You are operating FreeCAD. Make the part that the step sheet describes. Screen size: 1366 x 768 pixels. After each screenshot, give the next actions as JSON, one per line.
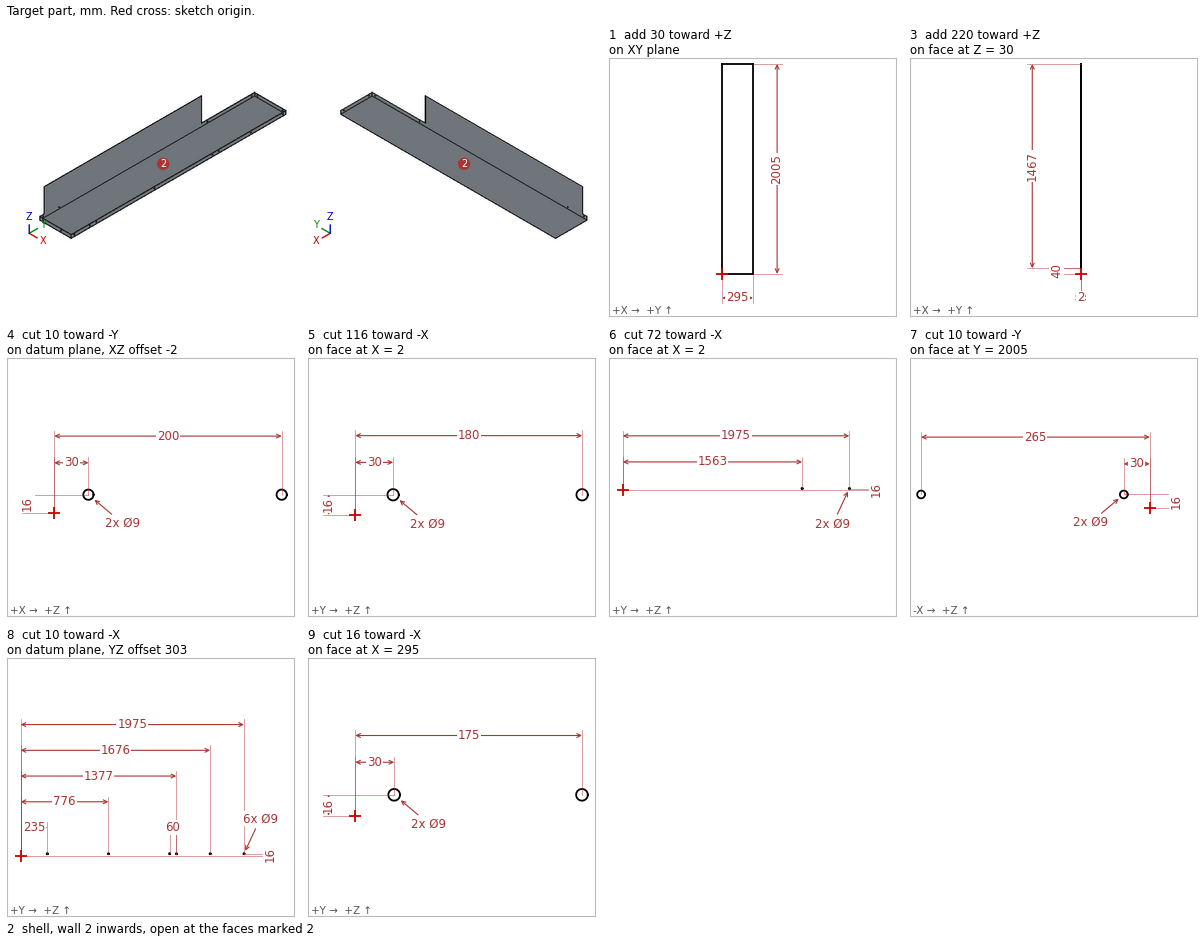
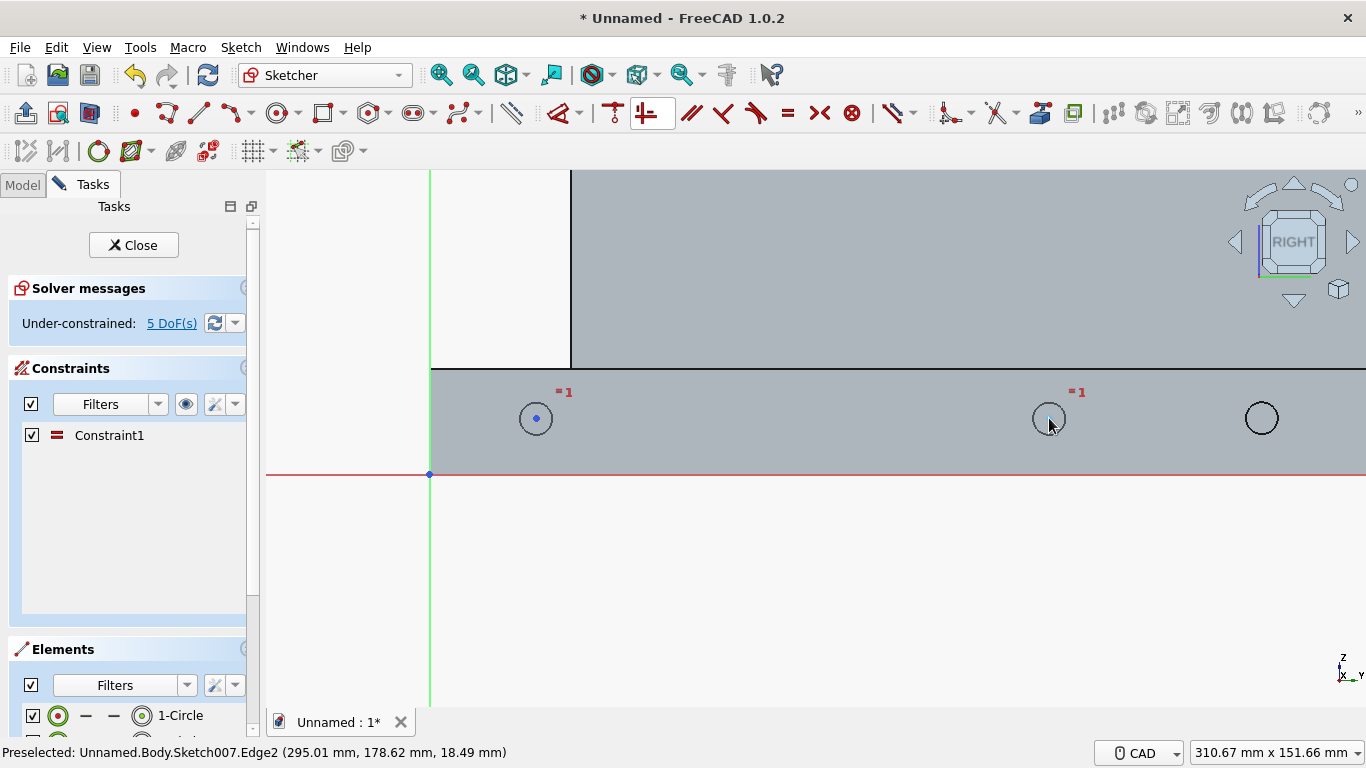
{"action": "left_click", "coordinate": [536, 419]}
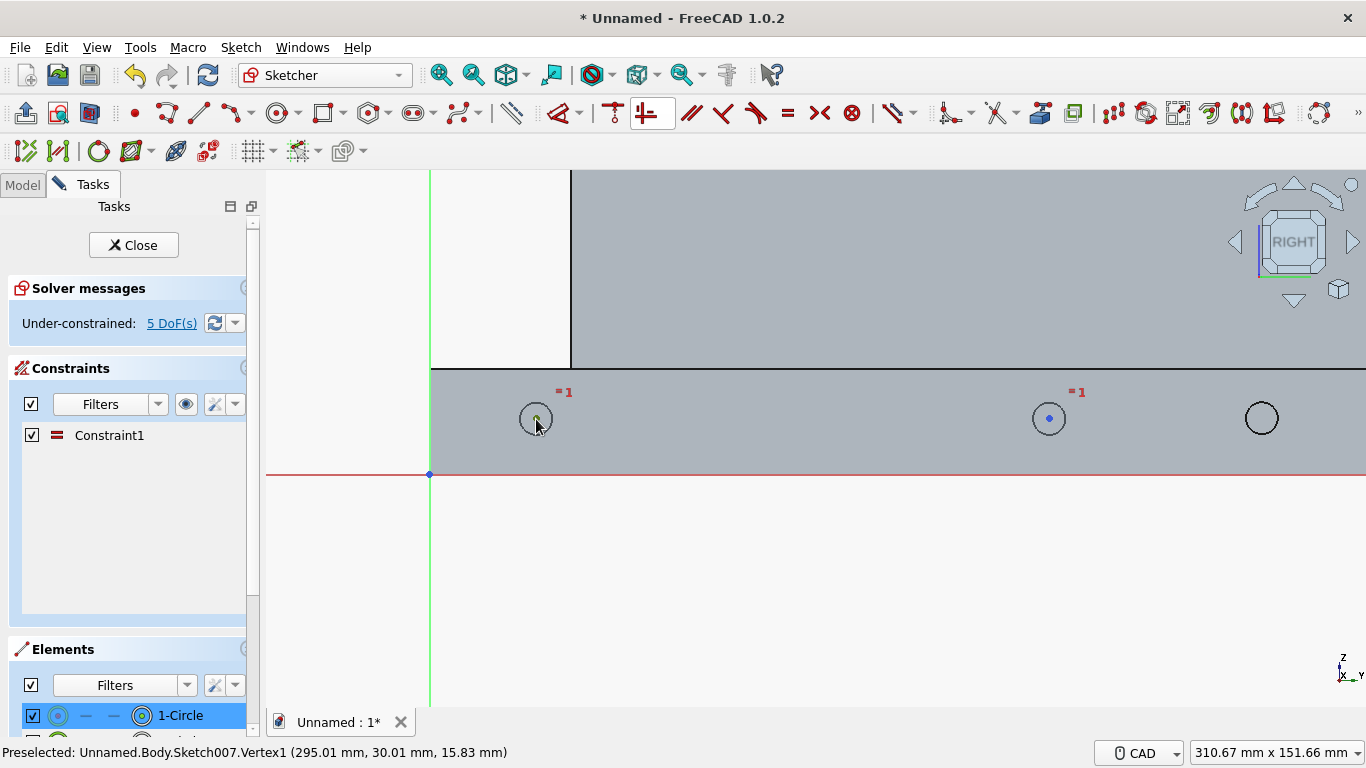
{"action": "left_click", "coordinate": [1049, 419]}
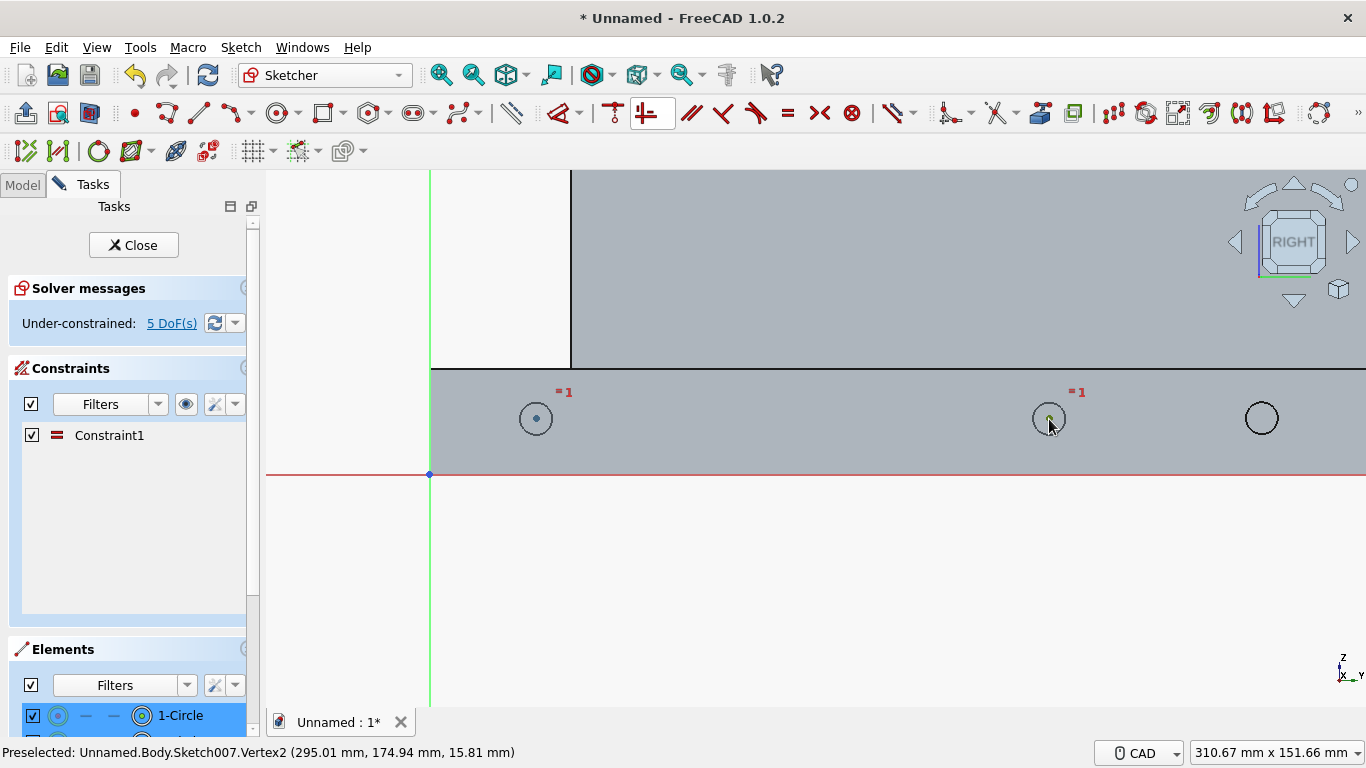
{"action": "left_click", "coordinate": [670, 114]}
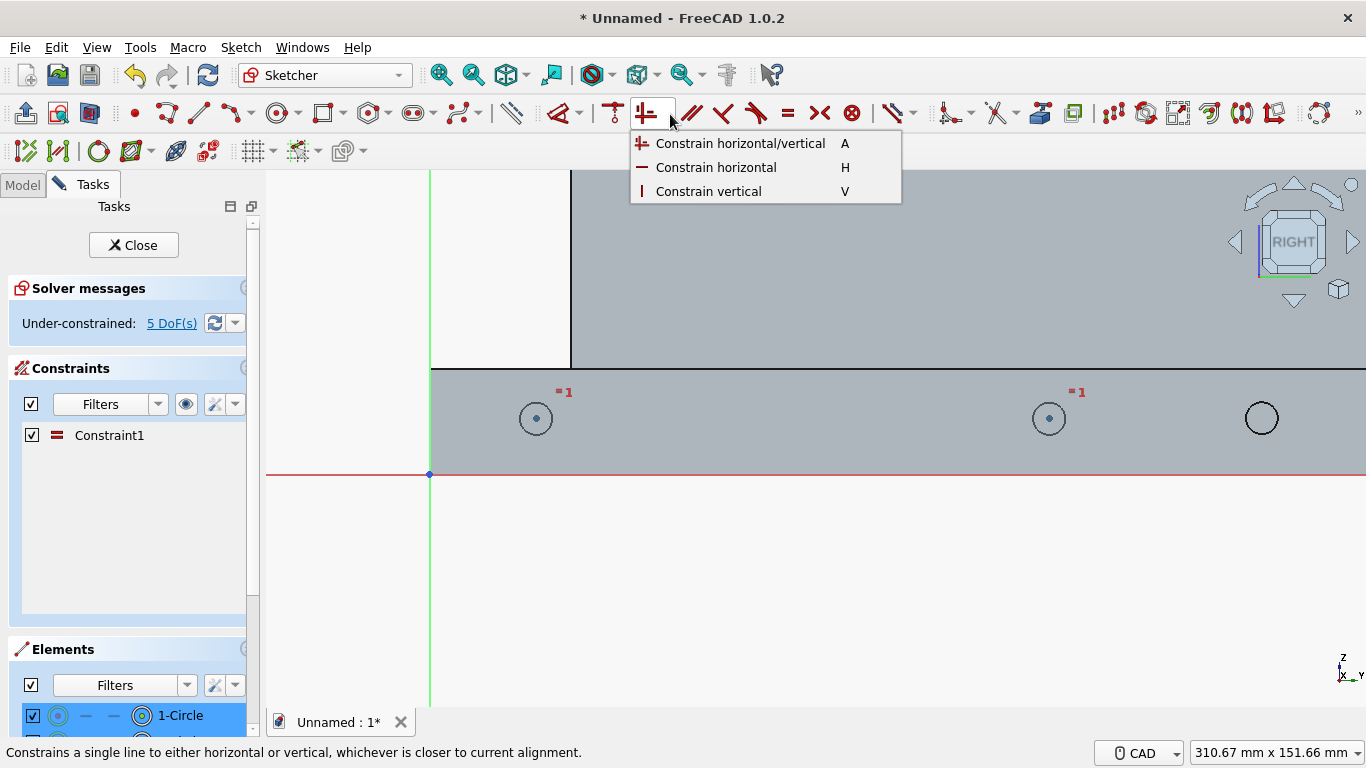
{"action": "left_click", "coordinate": [766, 167]}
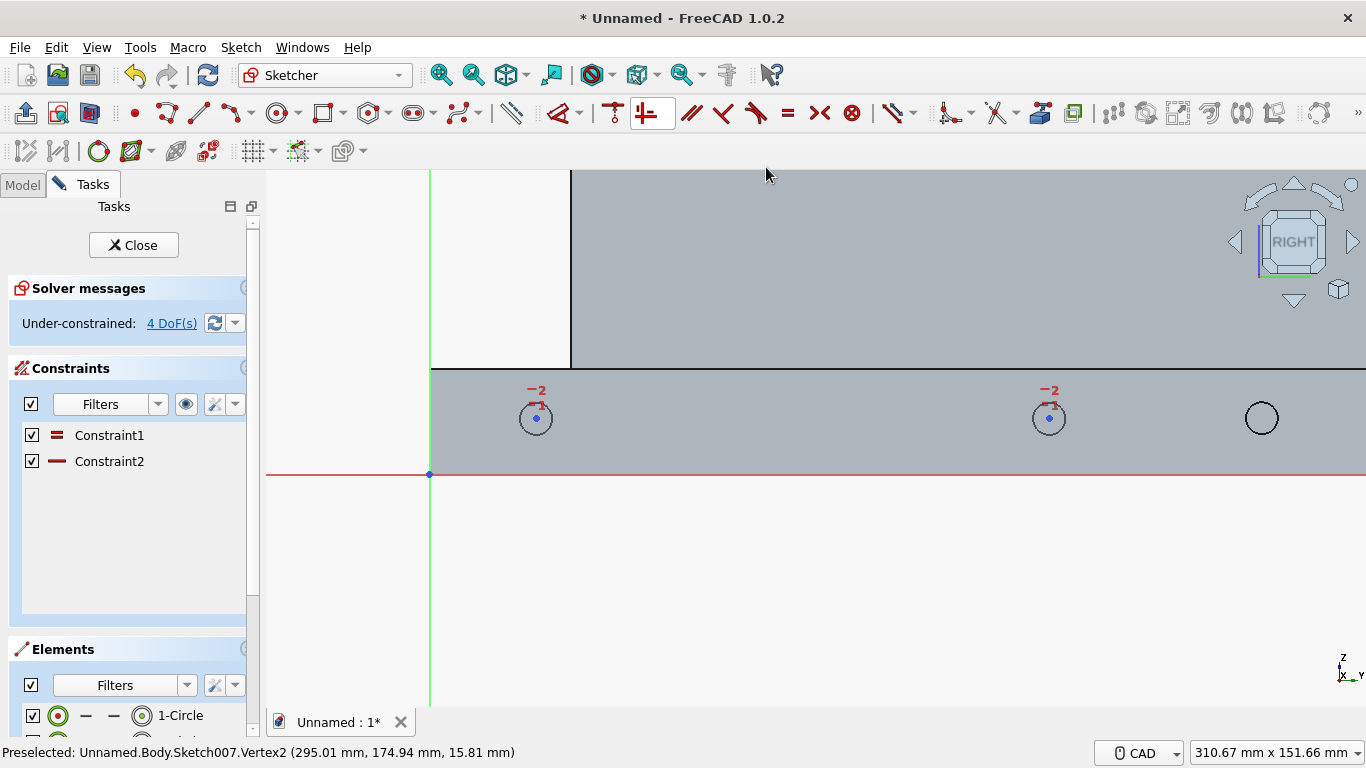
{"action": "left_click", "coordinate": [558, 114]}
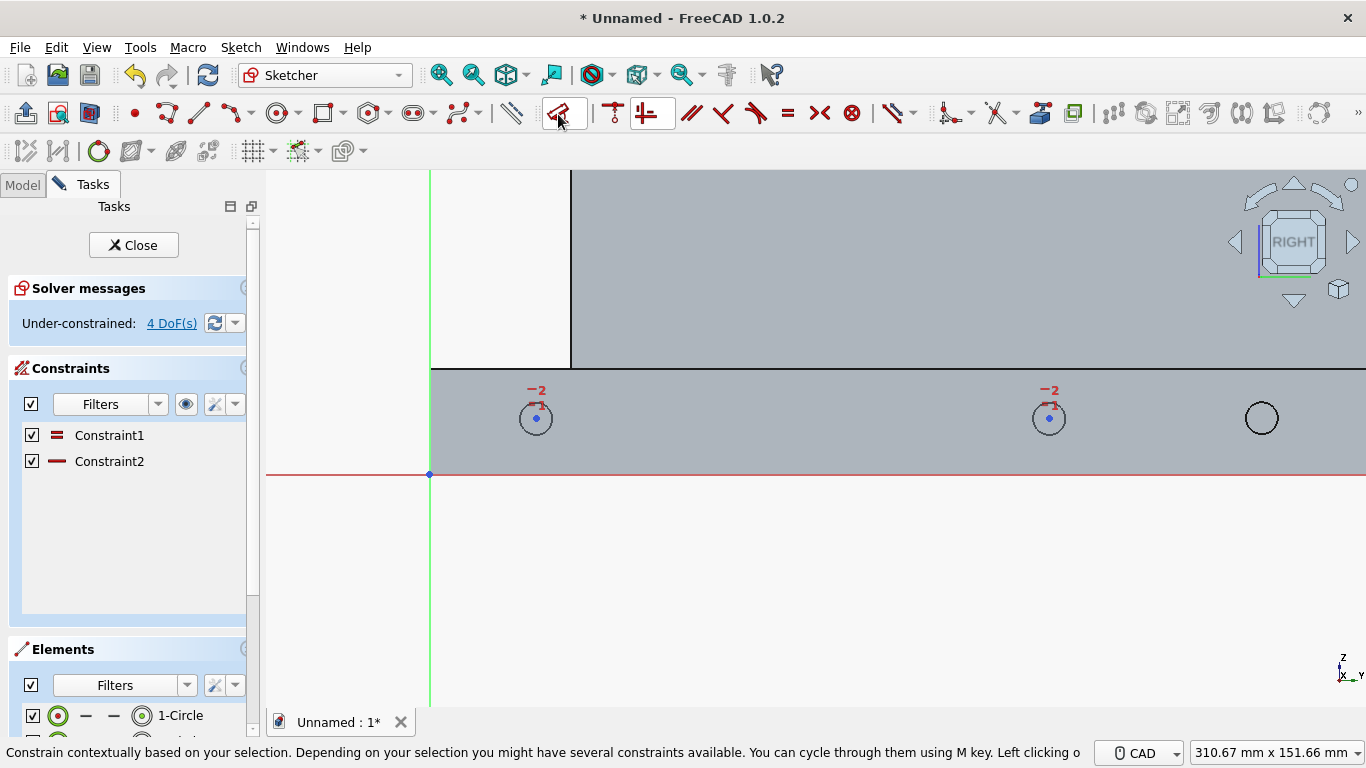
{"action": "scroll", "coordinate": [547, 407], "scroll_direction": "up", "scroll_amount": 2}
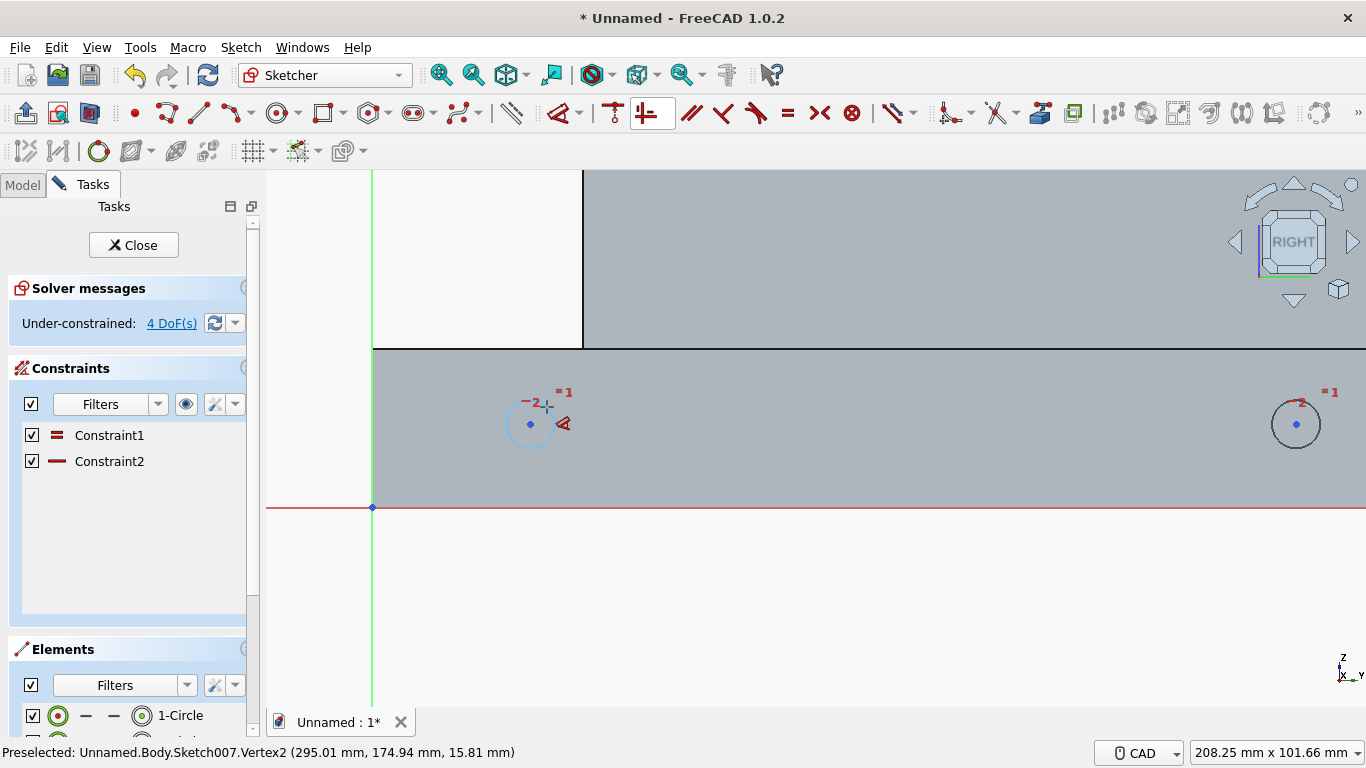
{"action": "left_click", "coordinate": [548, 407]}
{"action": "left_click", "coordinate": [571, 384]}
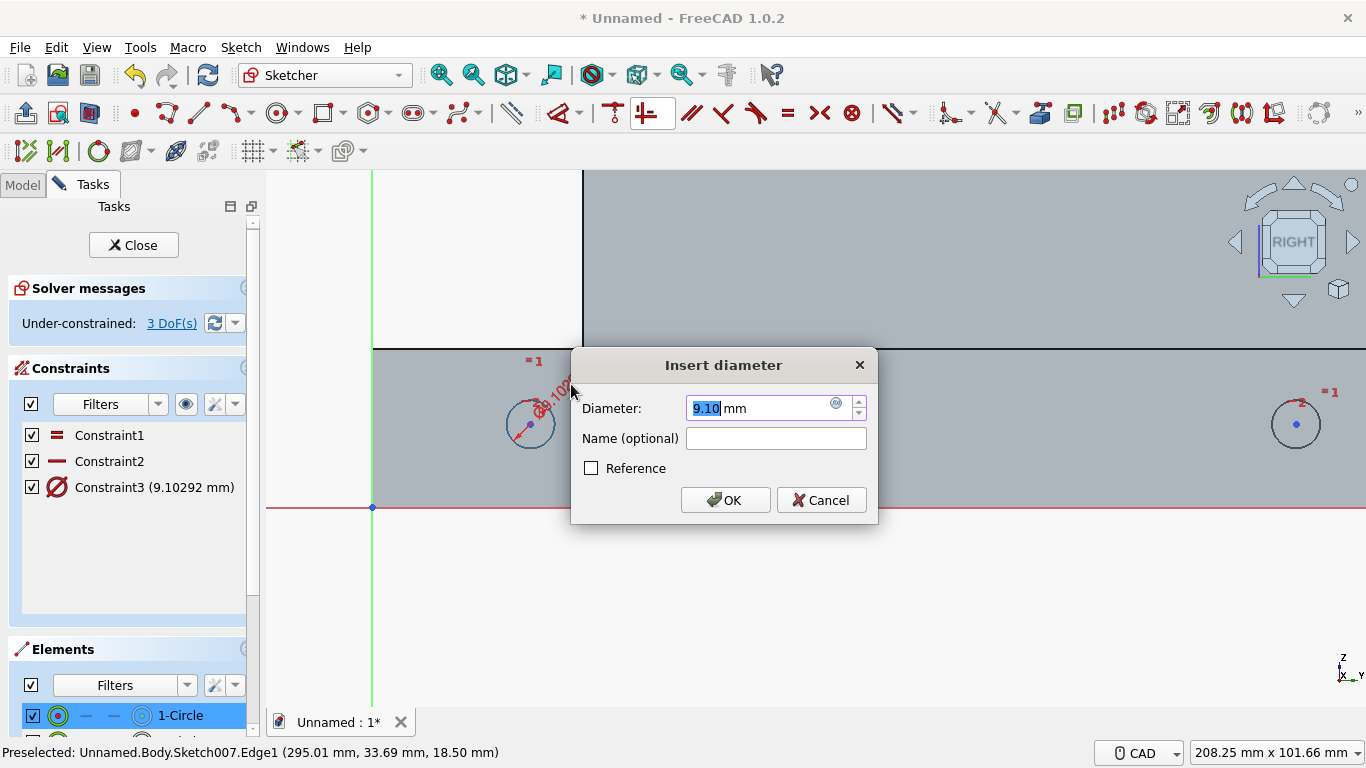
{"action": "type", "text": "9"}
{"action": "key", "text": "Return"}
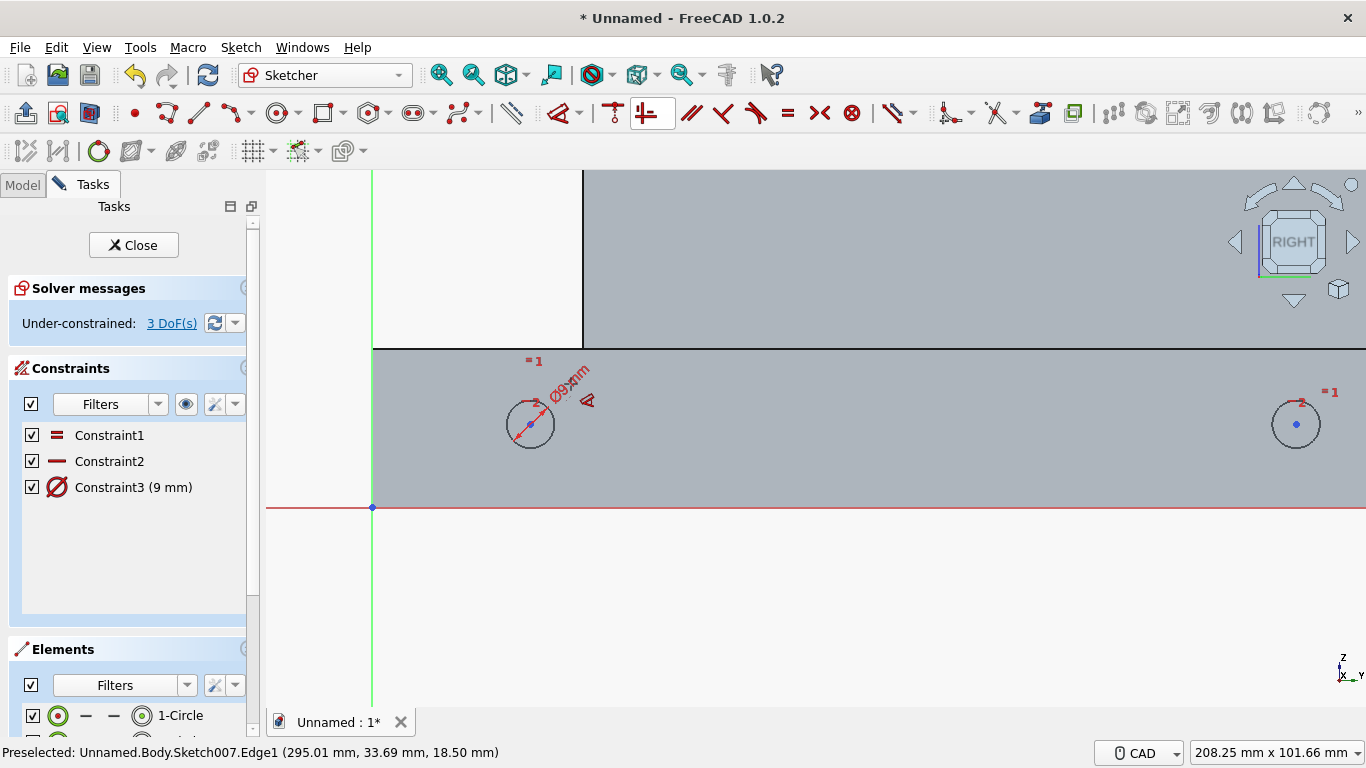
{"action": "left_click", "coordinate": [531, 424]}
{"action": "left_click", "coordinate": [451, 542]}